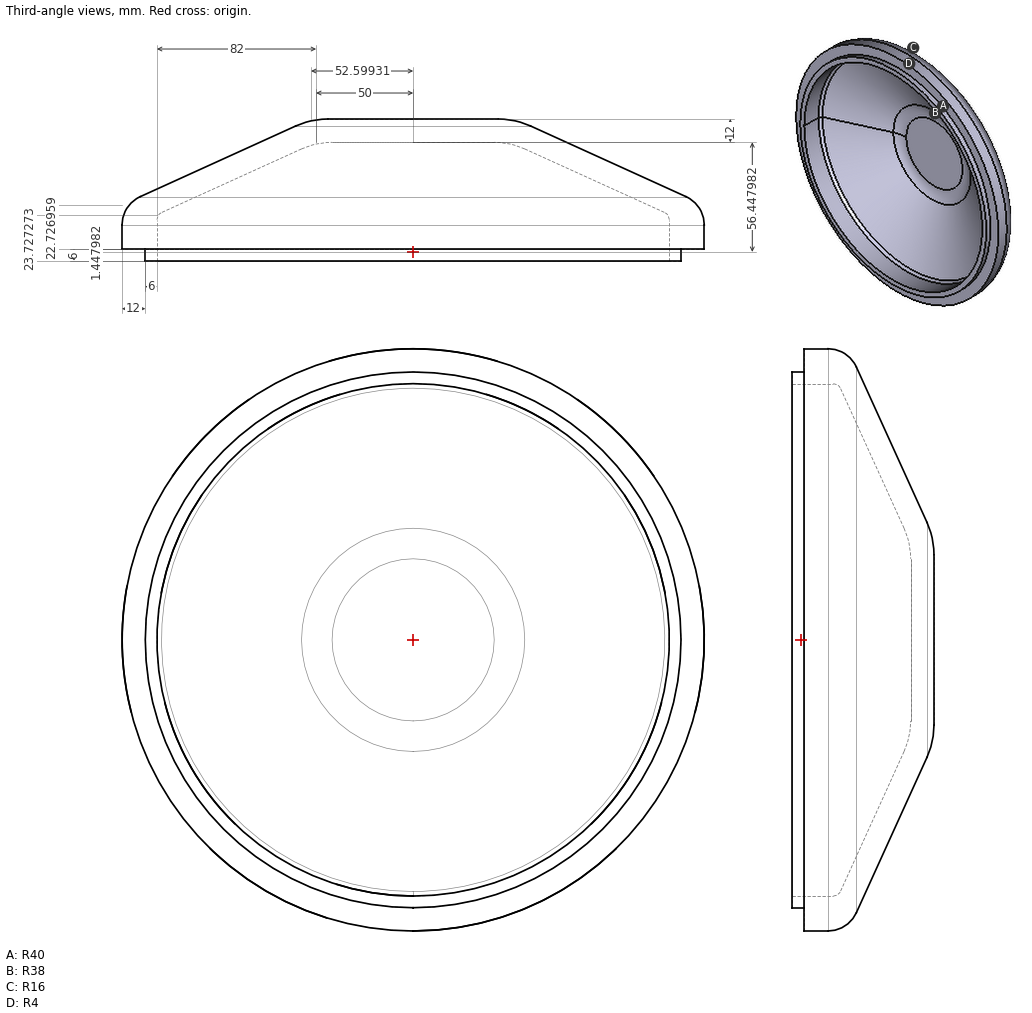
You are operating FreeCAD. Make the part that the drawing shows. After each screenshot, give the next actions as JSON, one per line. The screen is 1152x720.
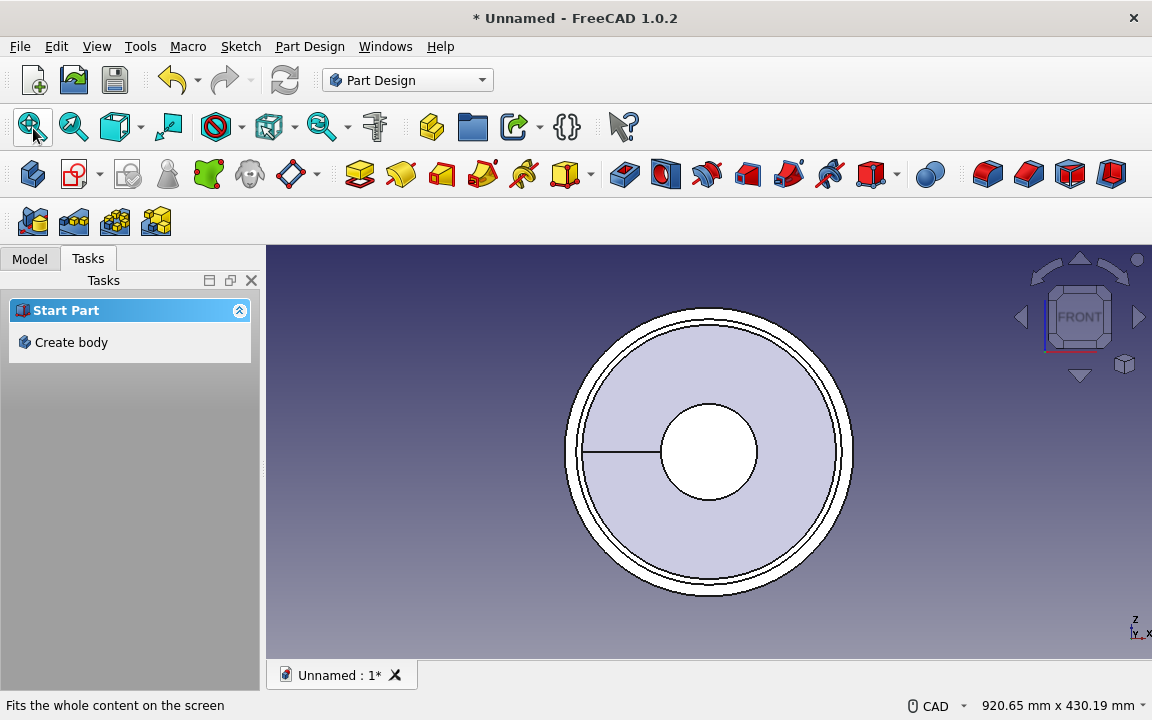
{"action": "key", "text": "3"}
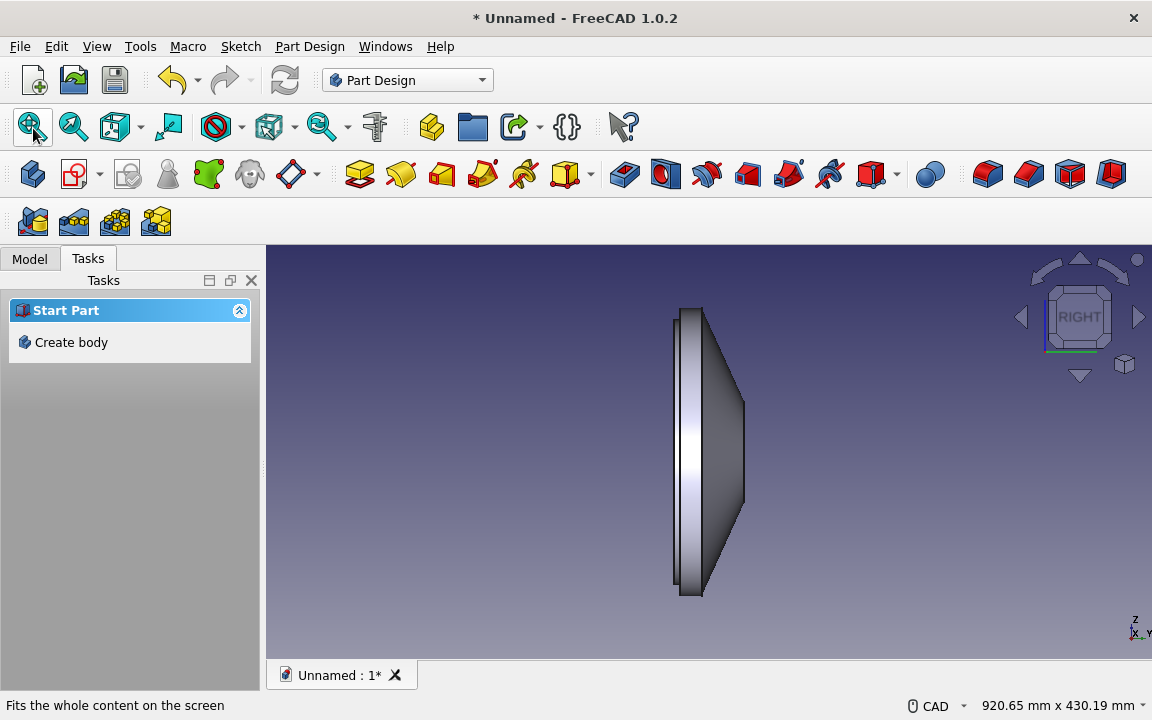
{"action": "key", "text": "5"}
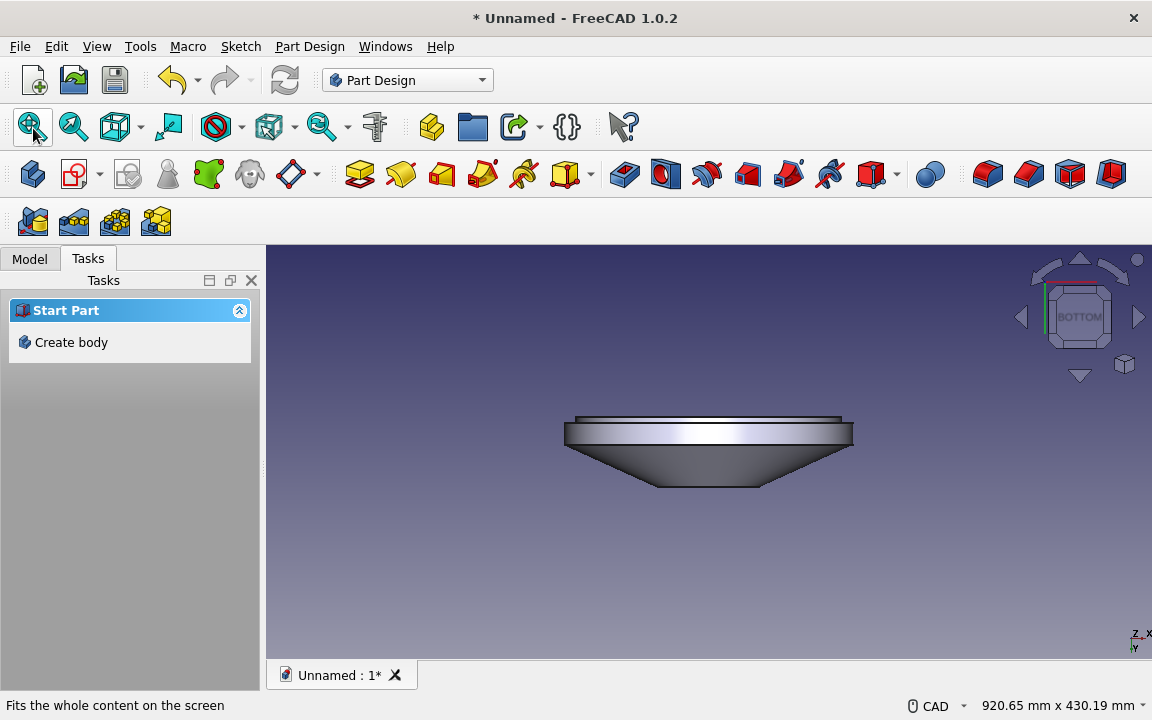
{"action": "left_click", "coordinate": [33, 128]}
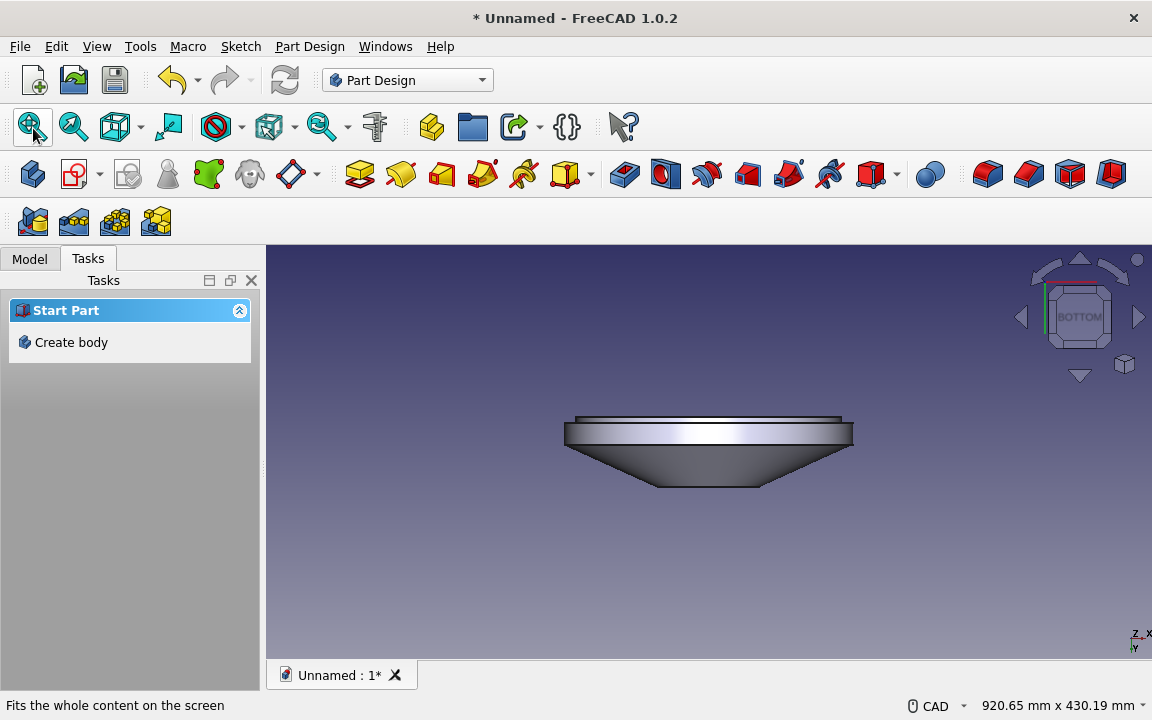
{"action": "key", "text": "4"}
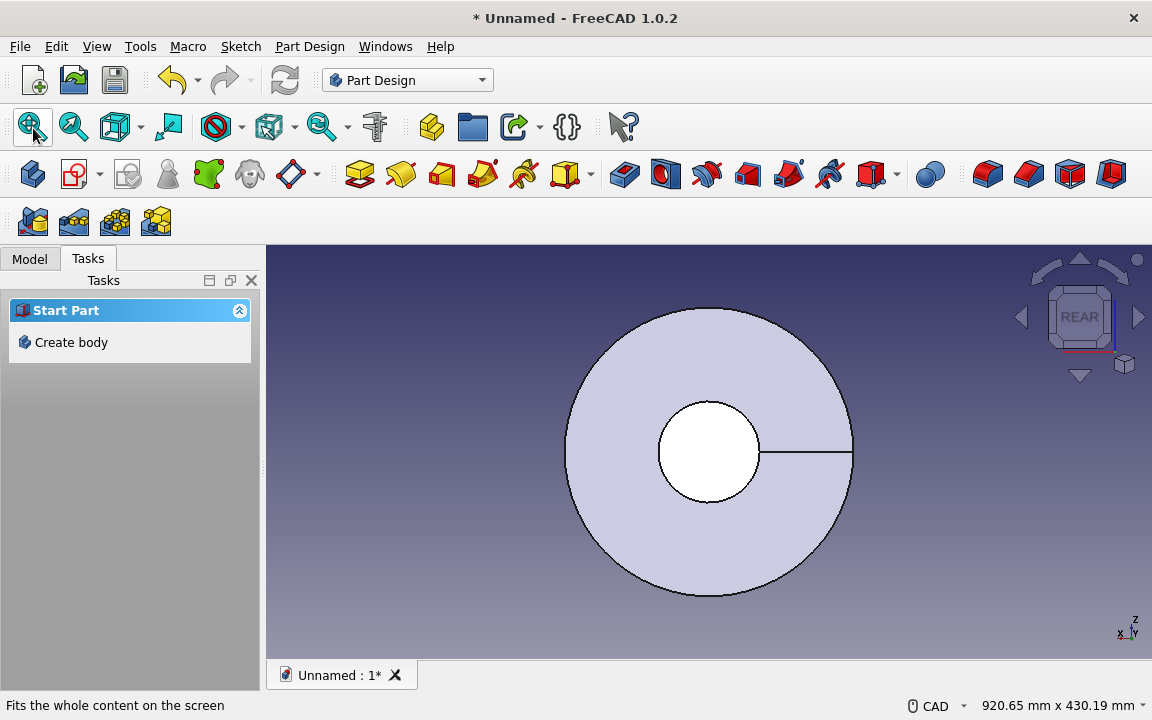
{"action": "left_click", "coordinate": [658, 451]}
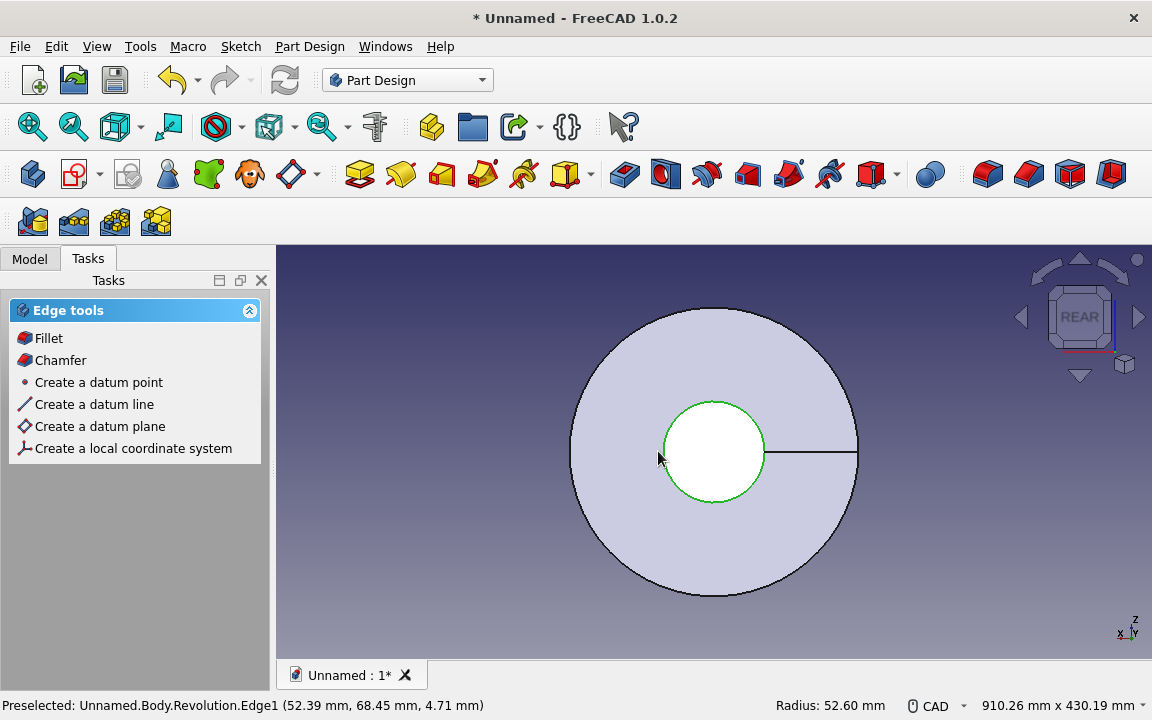
{"action": "left_click", "coordinate": [988, 174]}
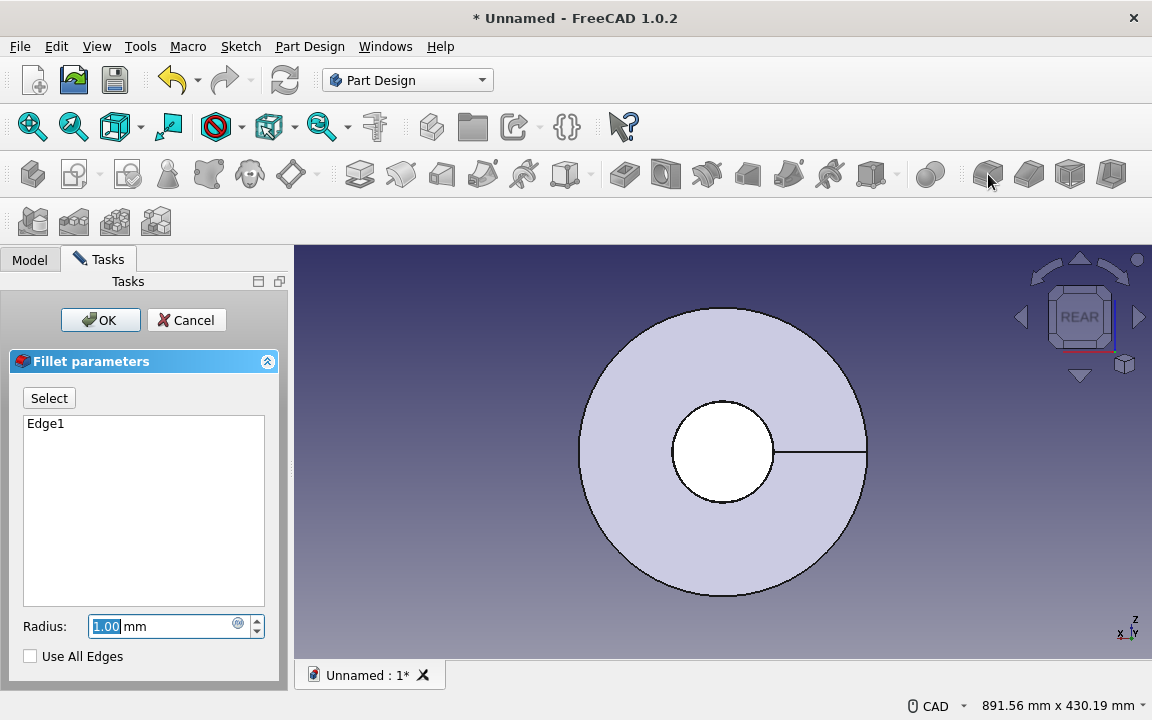
{"action": "type", "text": "40"}
{"action": "key", "text": "Tab"}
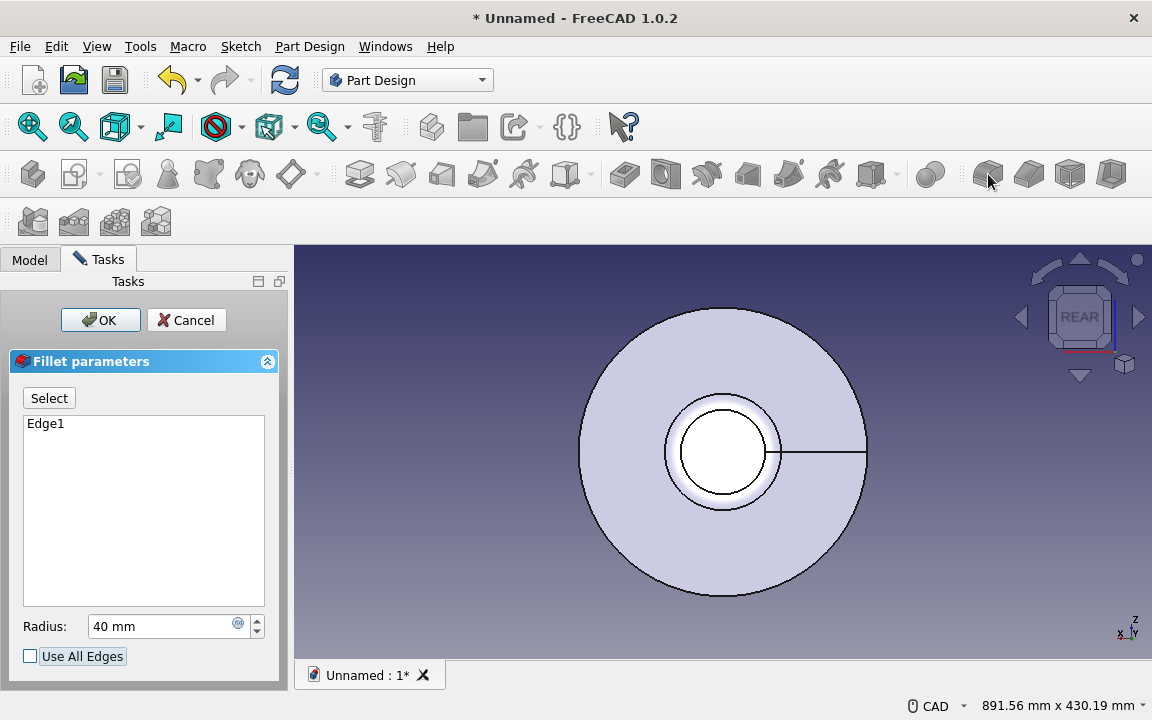
{"action": "left_click", "coordinate": [101, 320]}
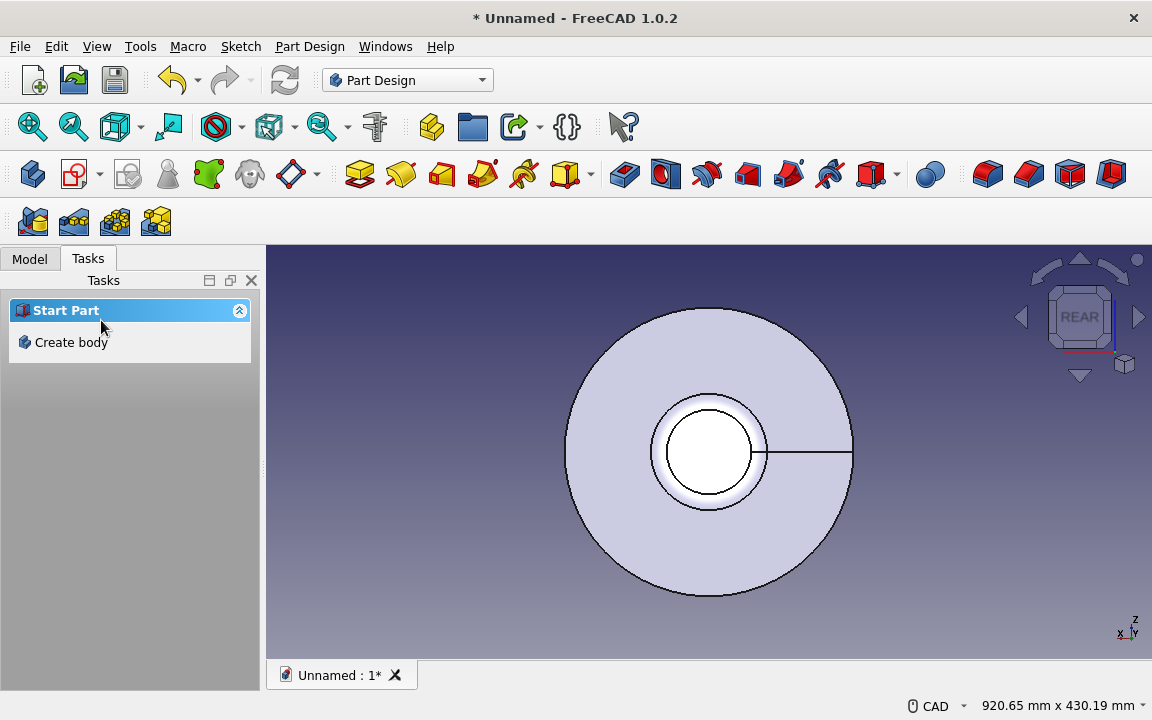
{"action": "key", "text": "0"}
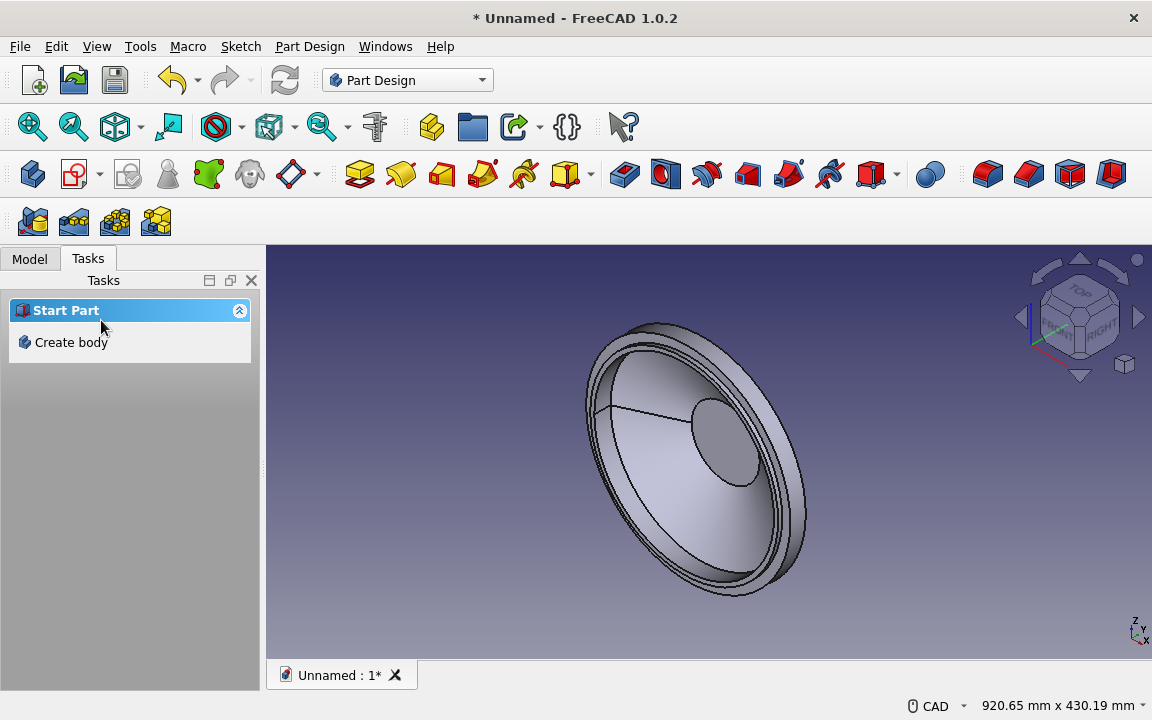
{"action": "left_click", "coordinate": [753, 480]}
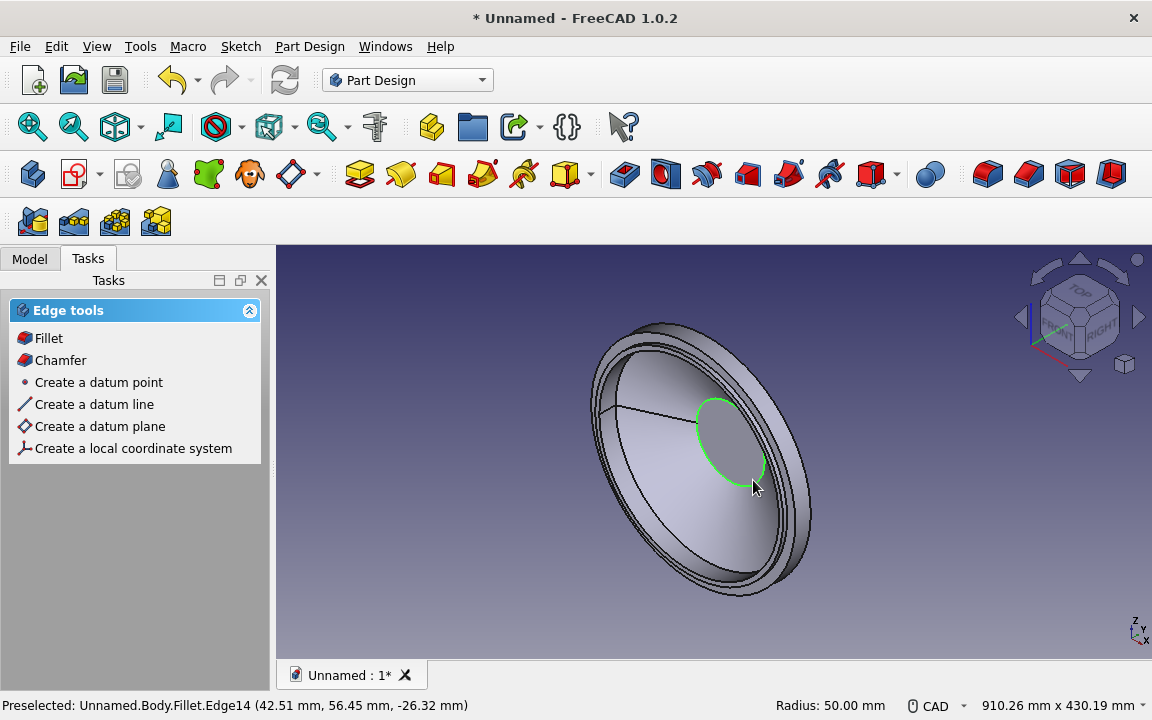
{"action": "left_click", "coordinate": [988, 174]}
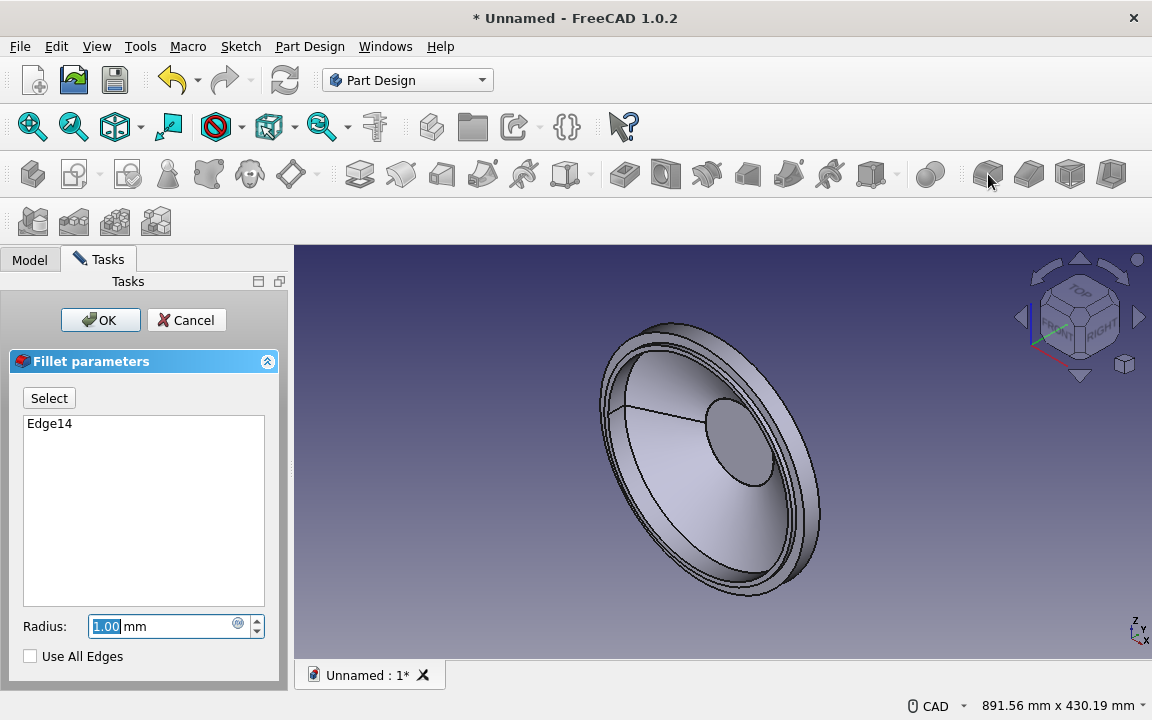
{"action": "type", "text": "38"}
{"action": "key", "text": "Tab"}